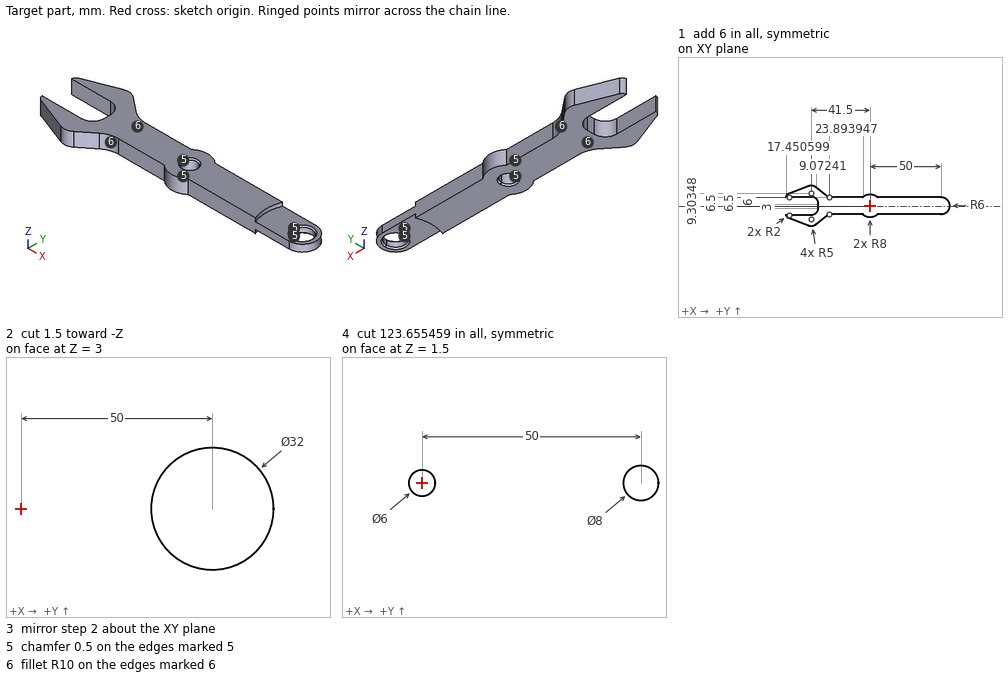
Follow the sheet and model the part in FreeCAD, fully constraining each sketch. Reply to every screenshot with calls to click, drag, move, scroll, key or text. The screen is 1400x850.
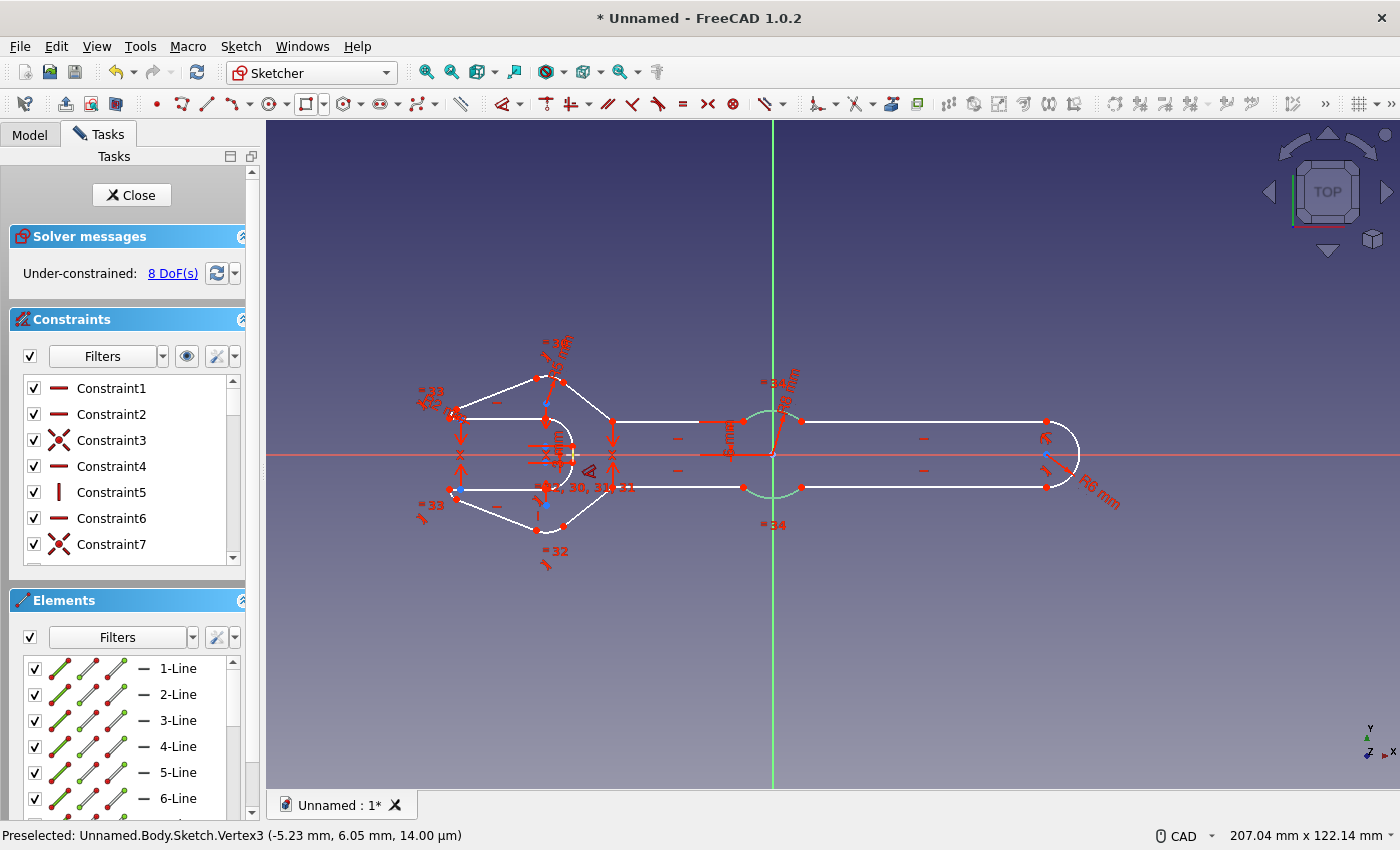
click(1046, 422)
click(910, 388)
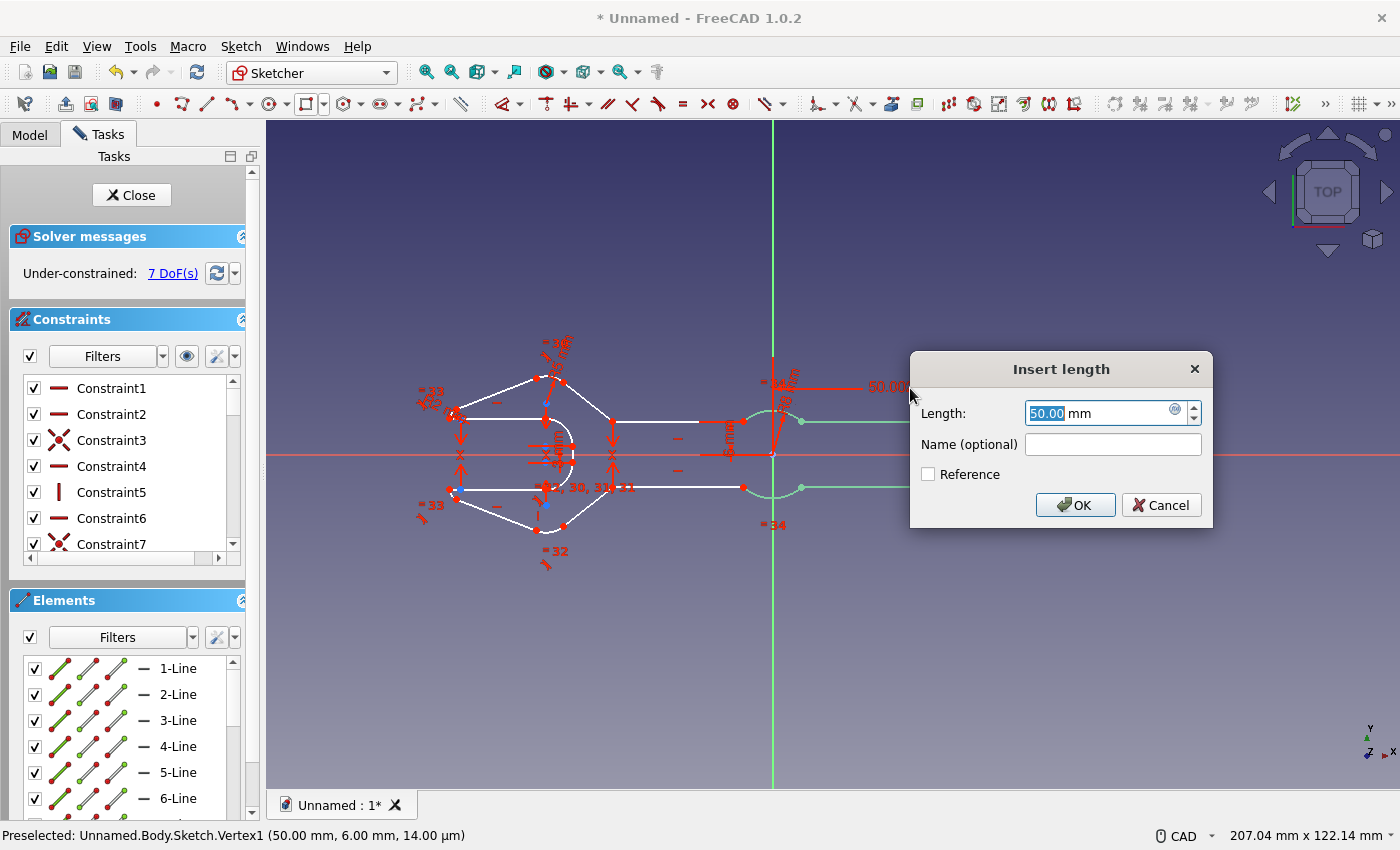
text(50)
key(Return)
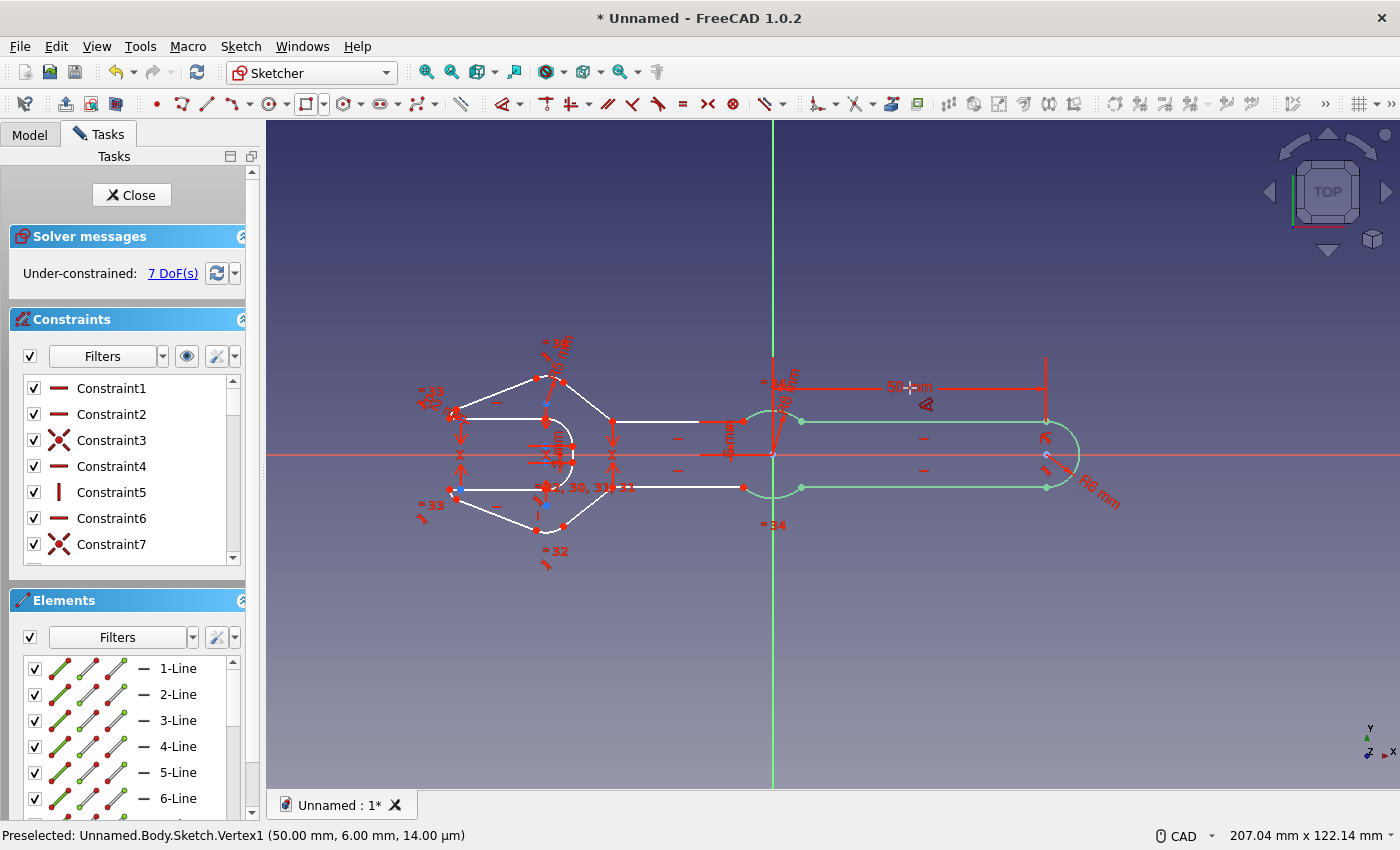
click(450, 419)
click(416, 437)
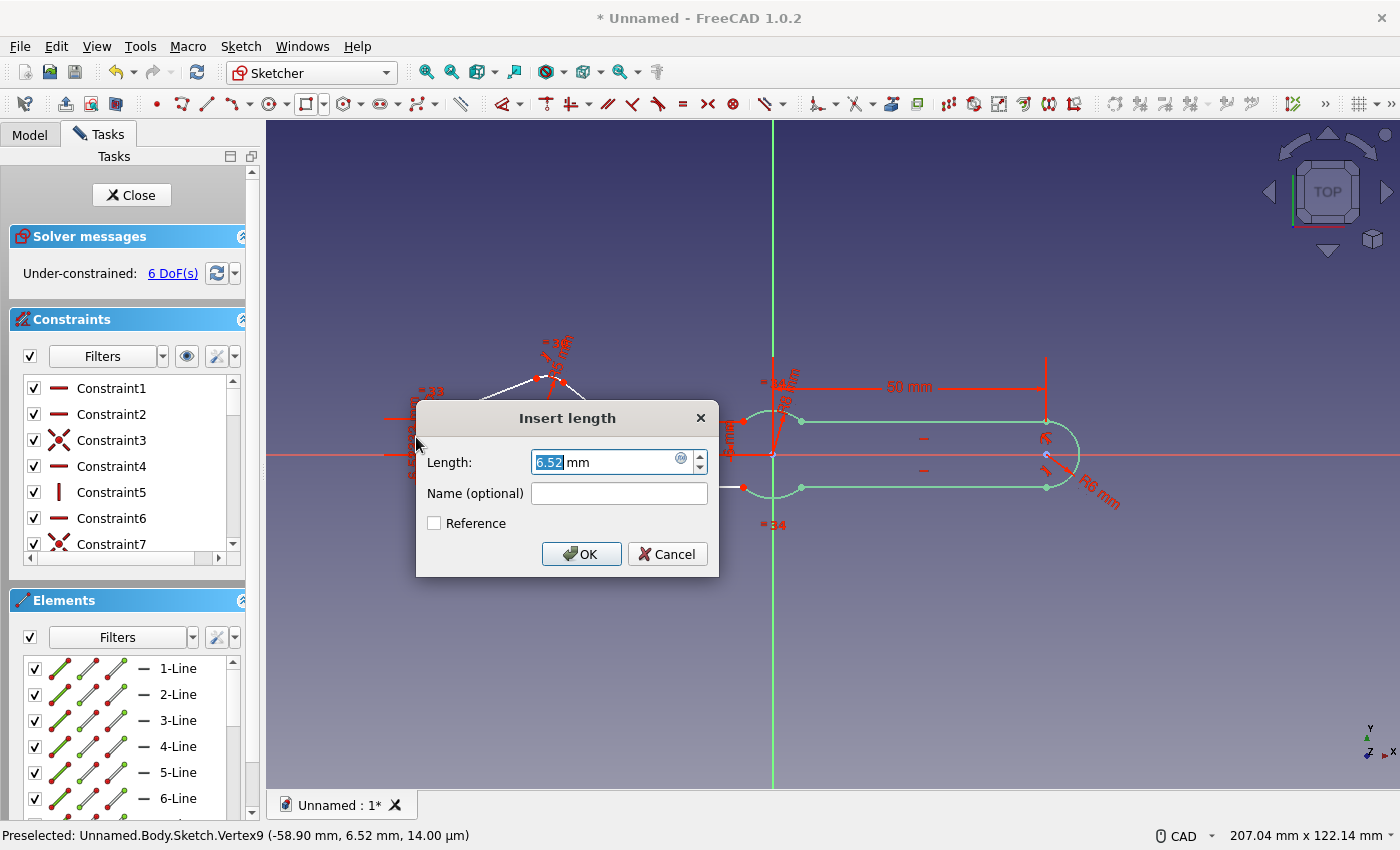
text(6.5)
key(Return)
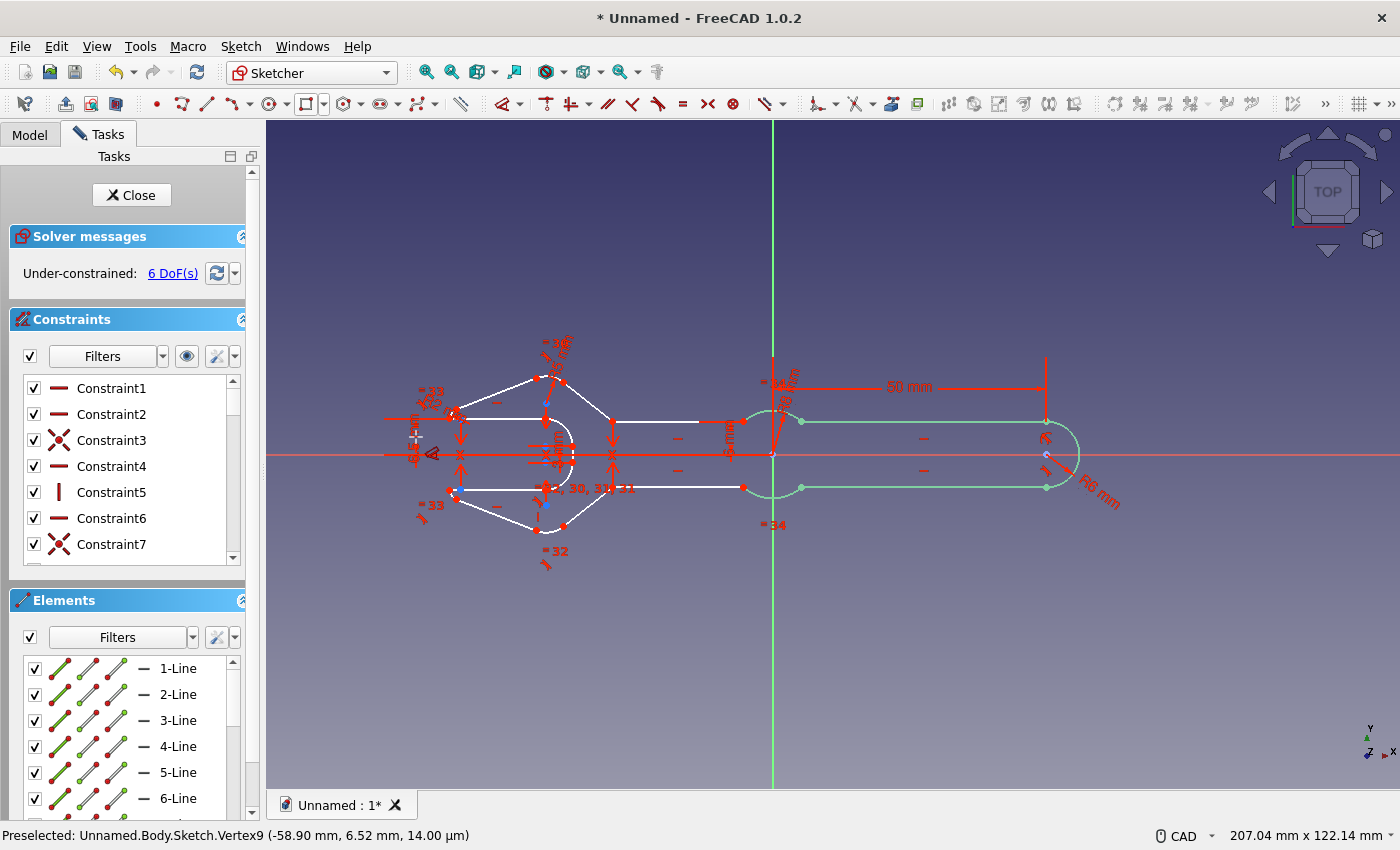
click(461, 419)
click(807, 437)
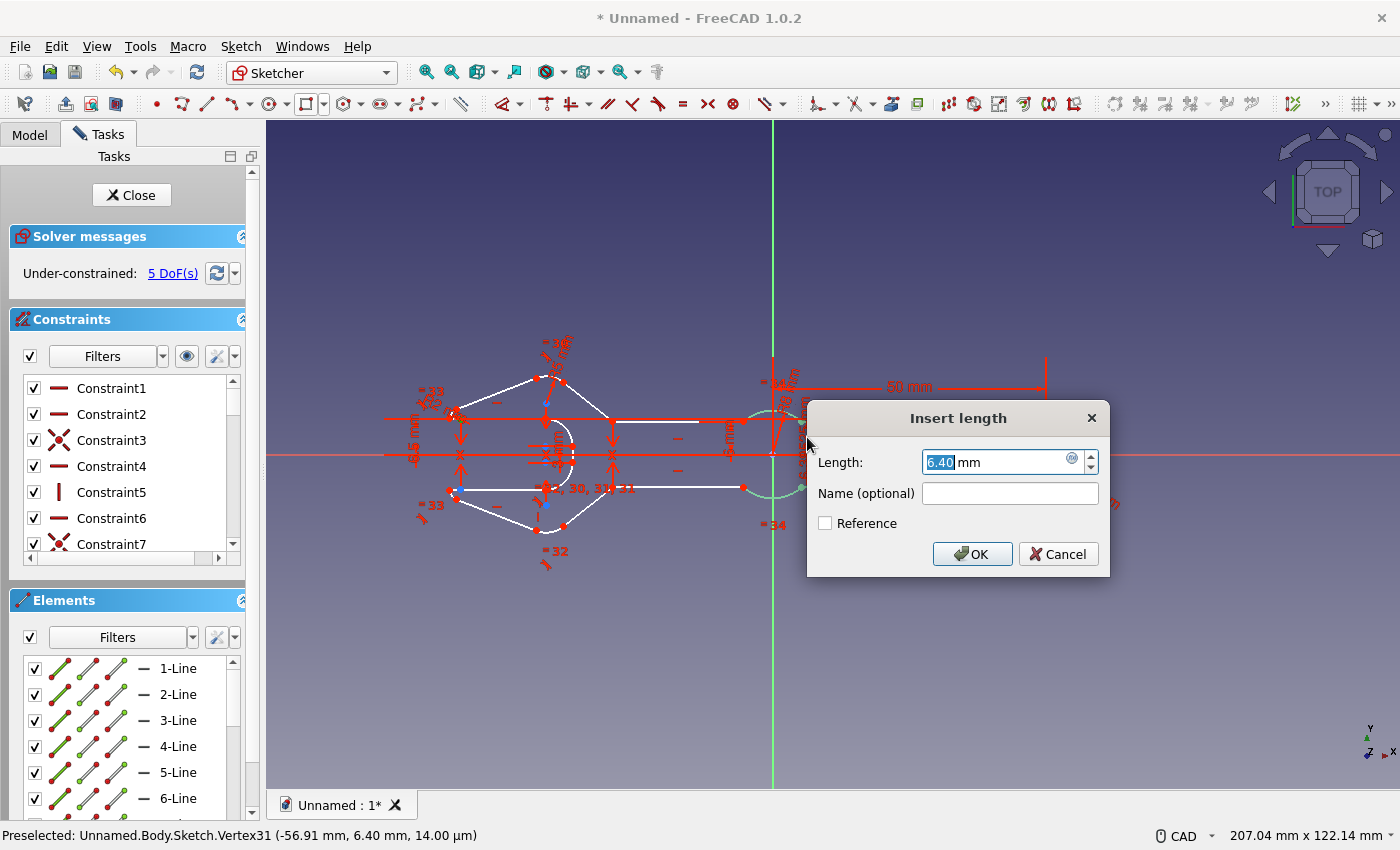
text(6.5)
key(Return)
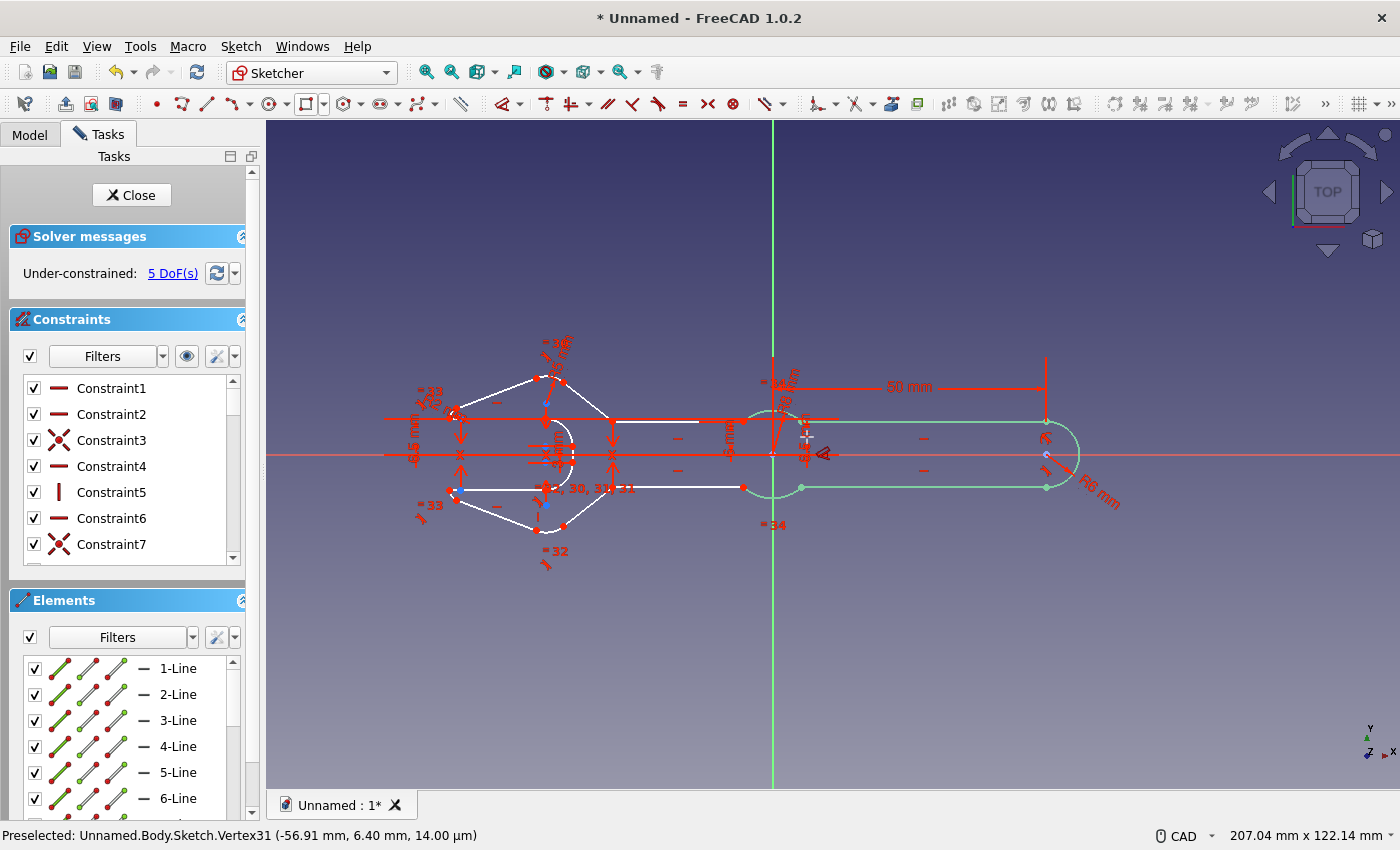
click(545, 419)
click(659, 385)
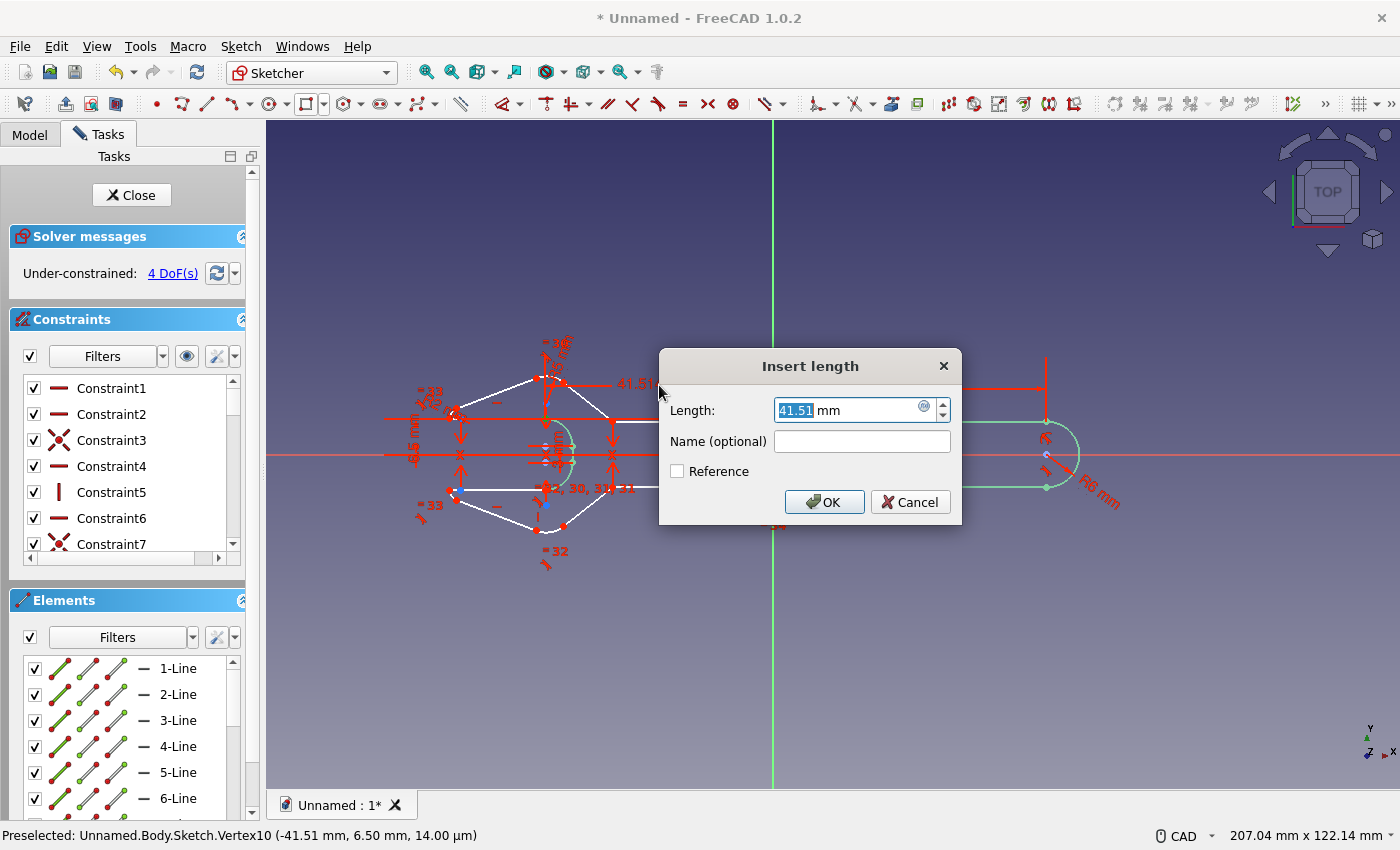
text(41.5)
key(Return)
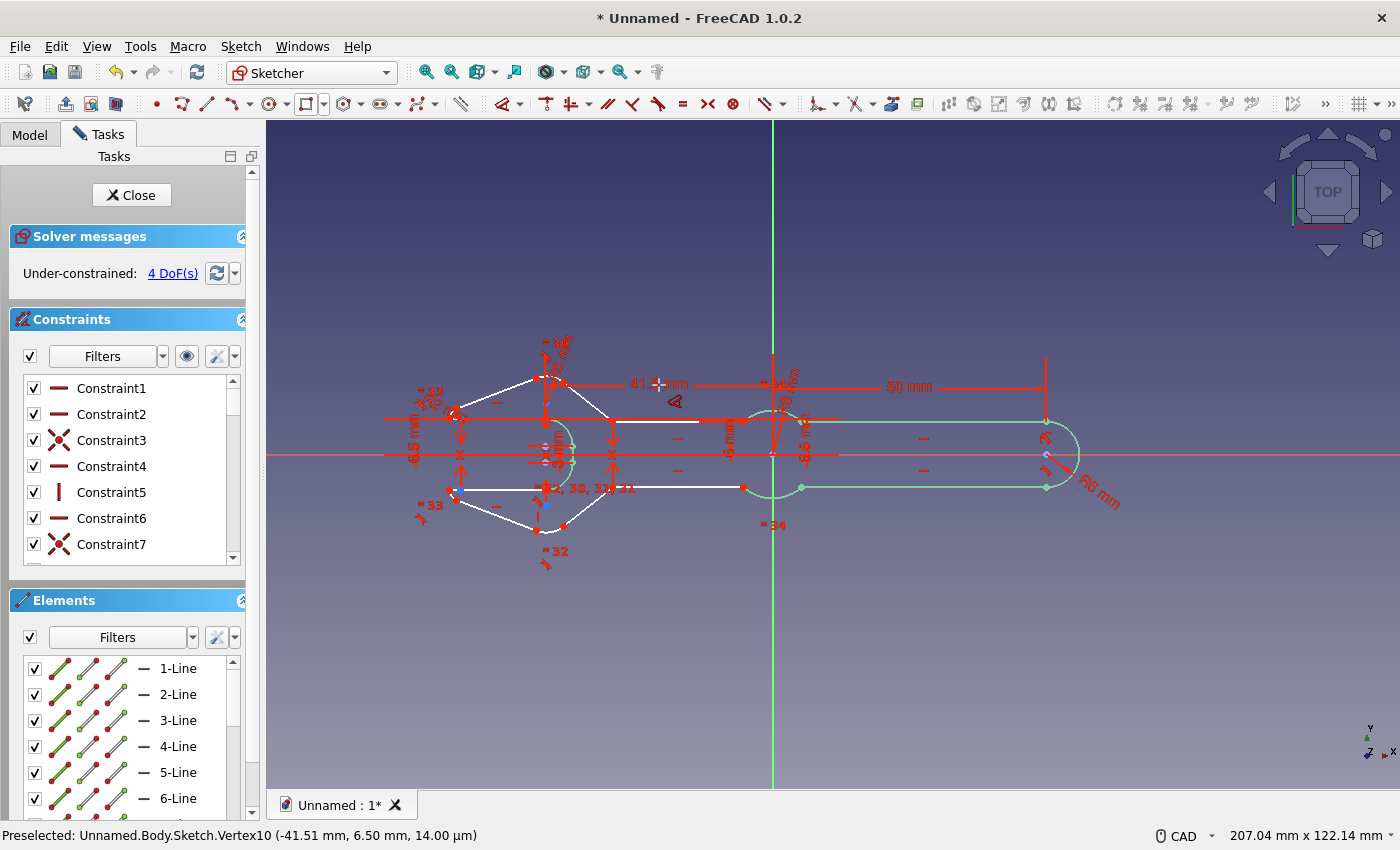
click(598, 410)
click(588, 324)